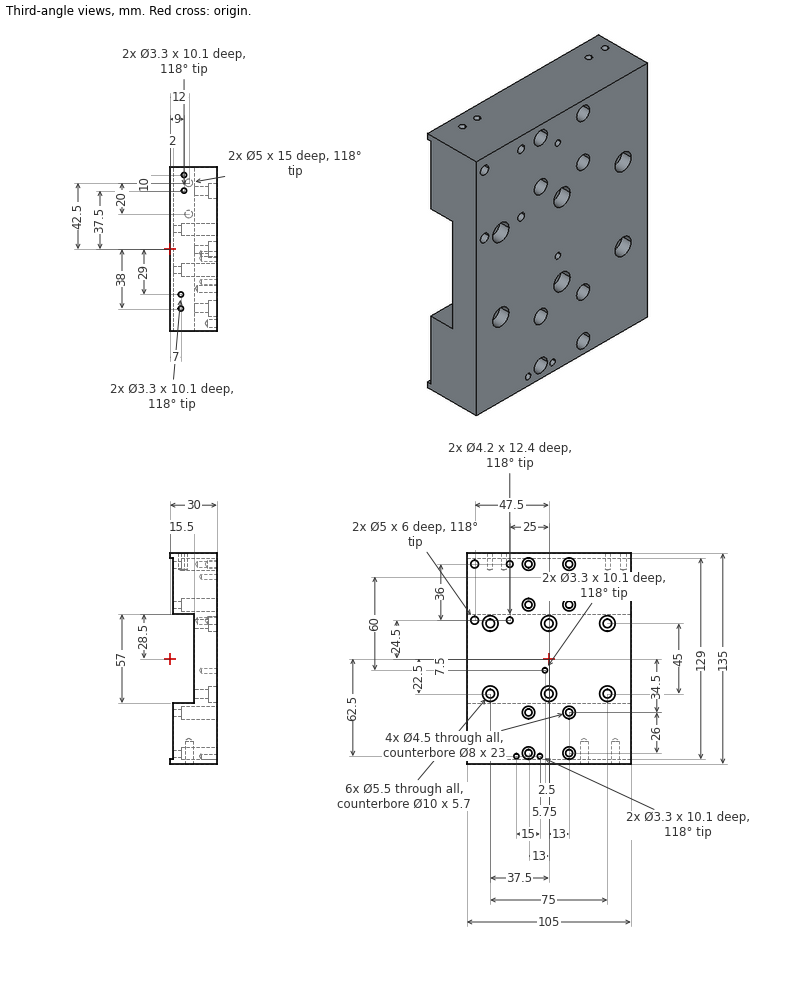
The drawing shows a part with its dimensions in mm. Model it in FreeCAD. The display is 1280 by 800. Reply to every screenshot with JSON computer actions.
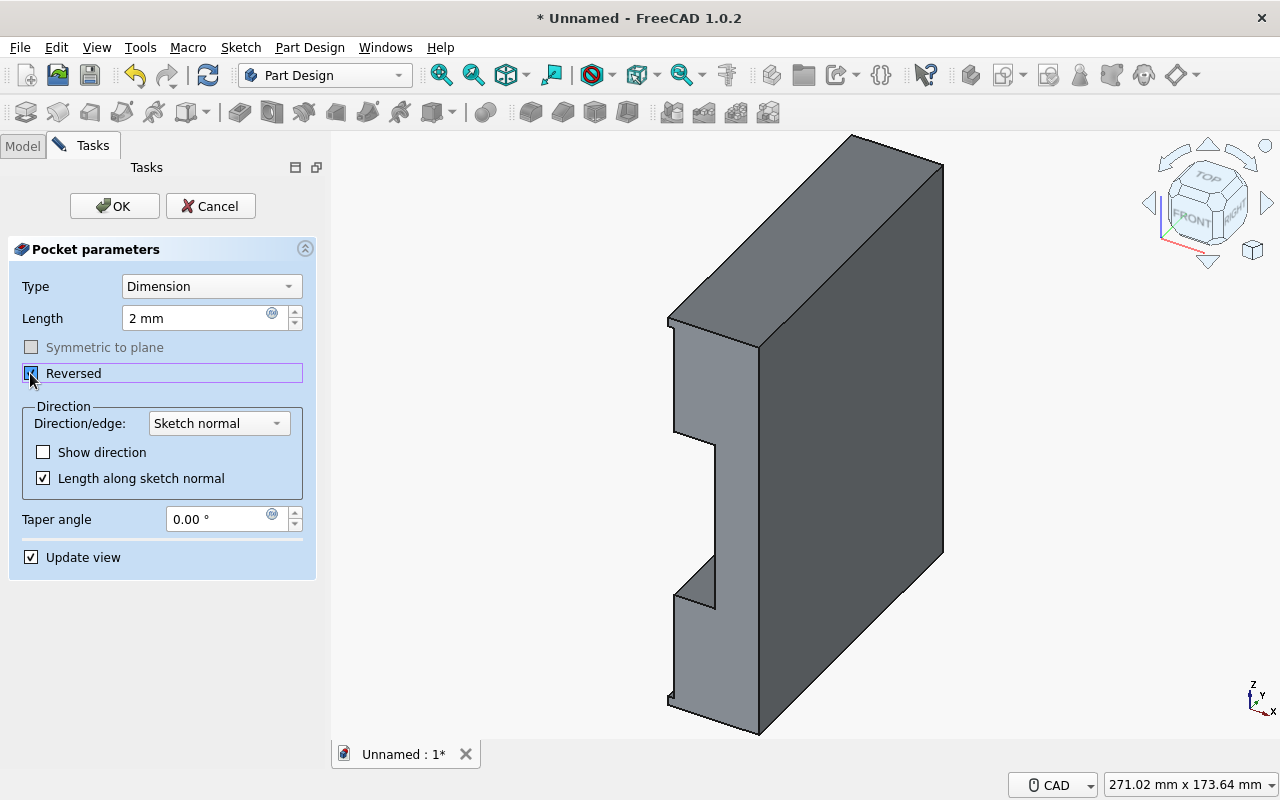
{"action": "left_click", "coordinate": [115, 206]}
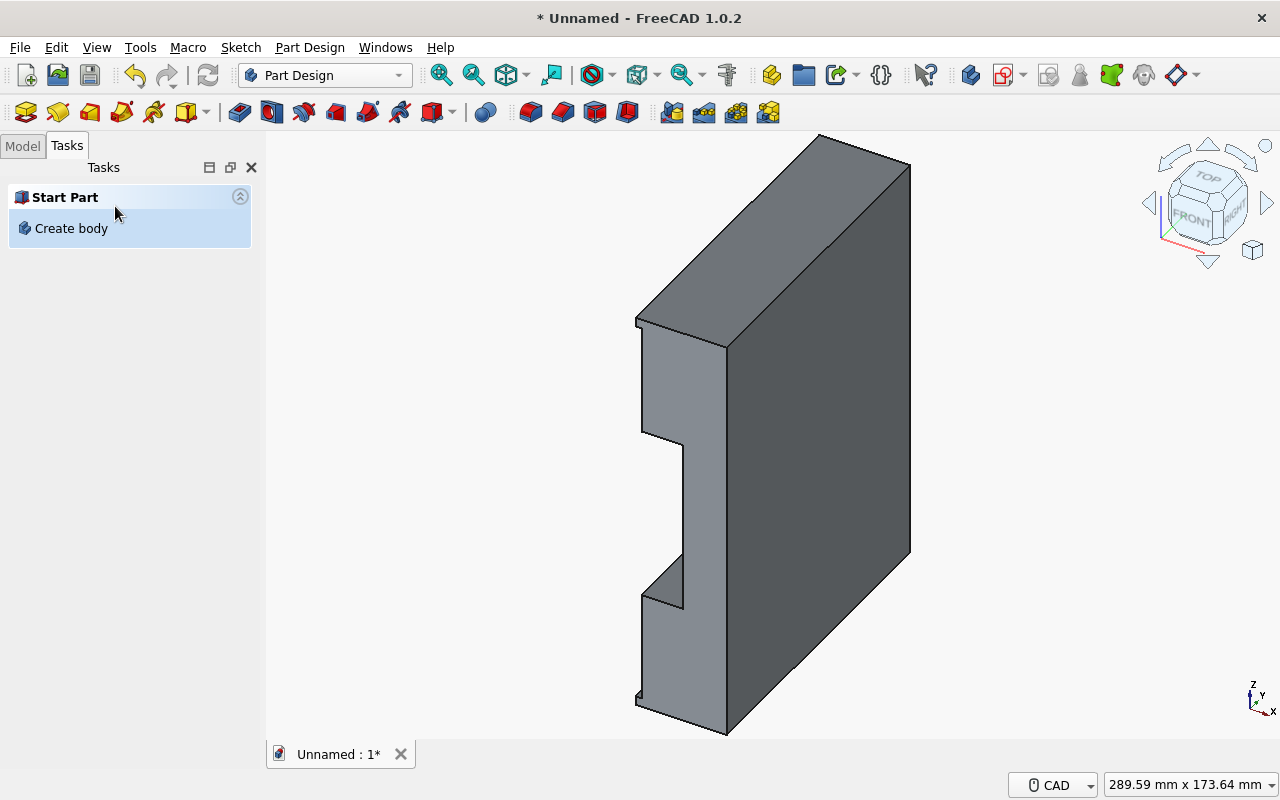
{"action": "left_click", "coordinate": [818, 449]}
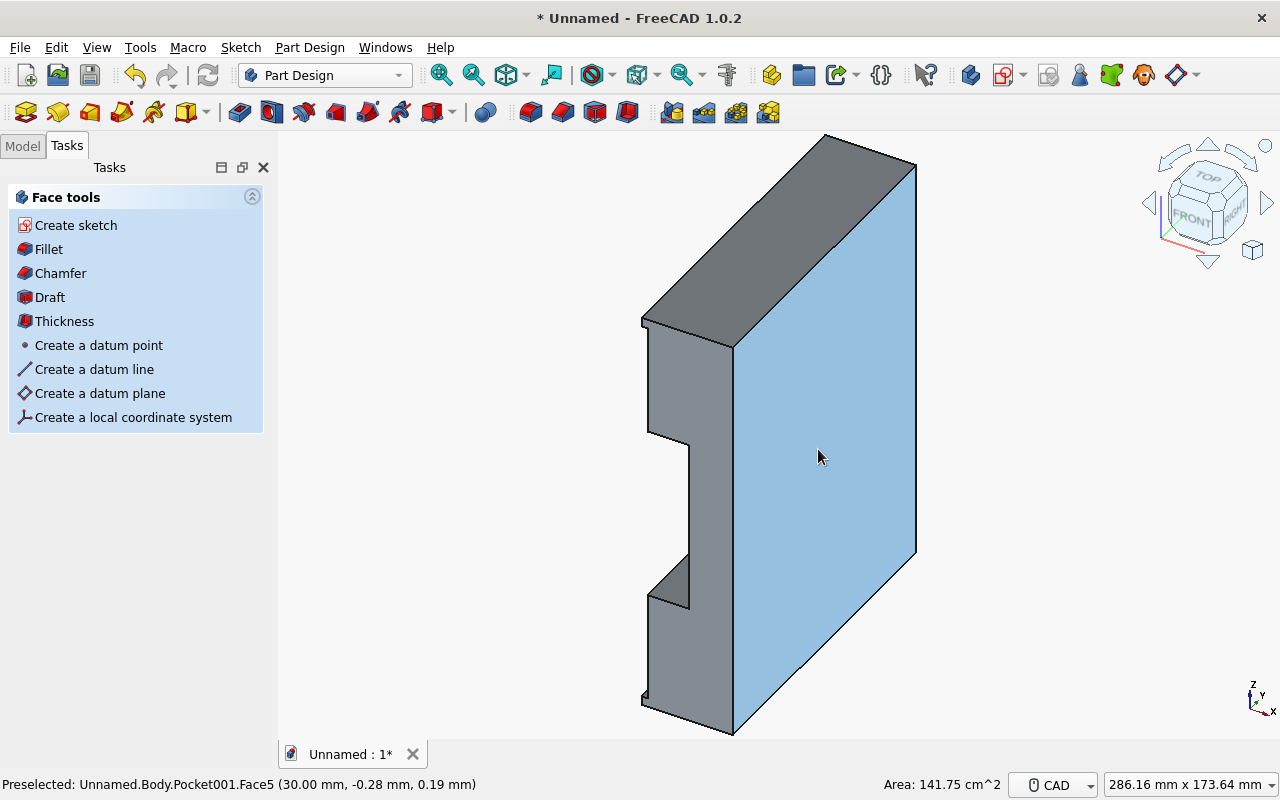
{"action": "left_click", "coordinate": [1004, 76]}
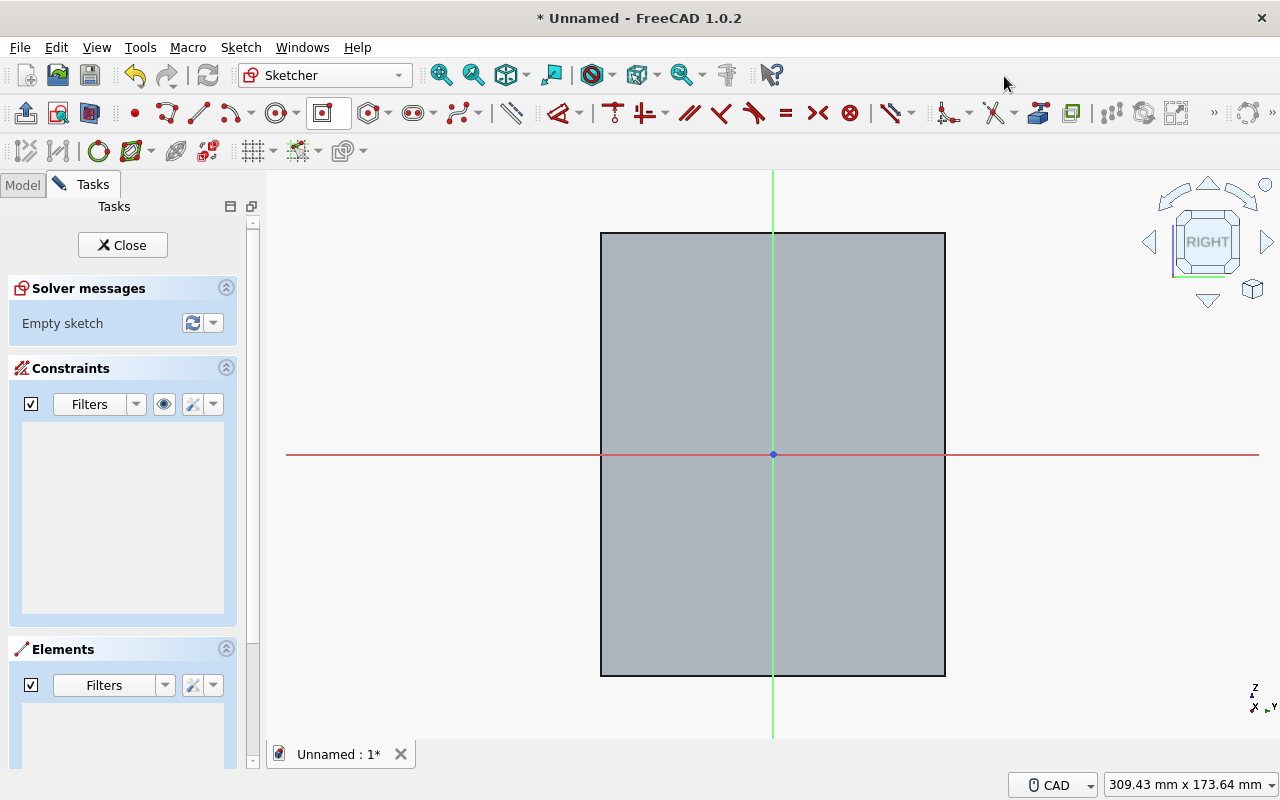
{"action": "scroll", "coordinate": [829, 454], "scroll_direction": "up", "scroll_amount": 4}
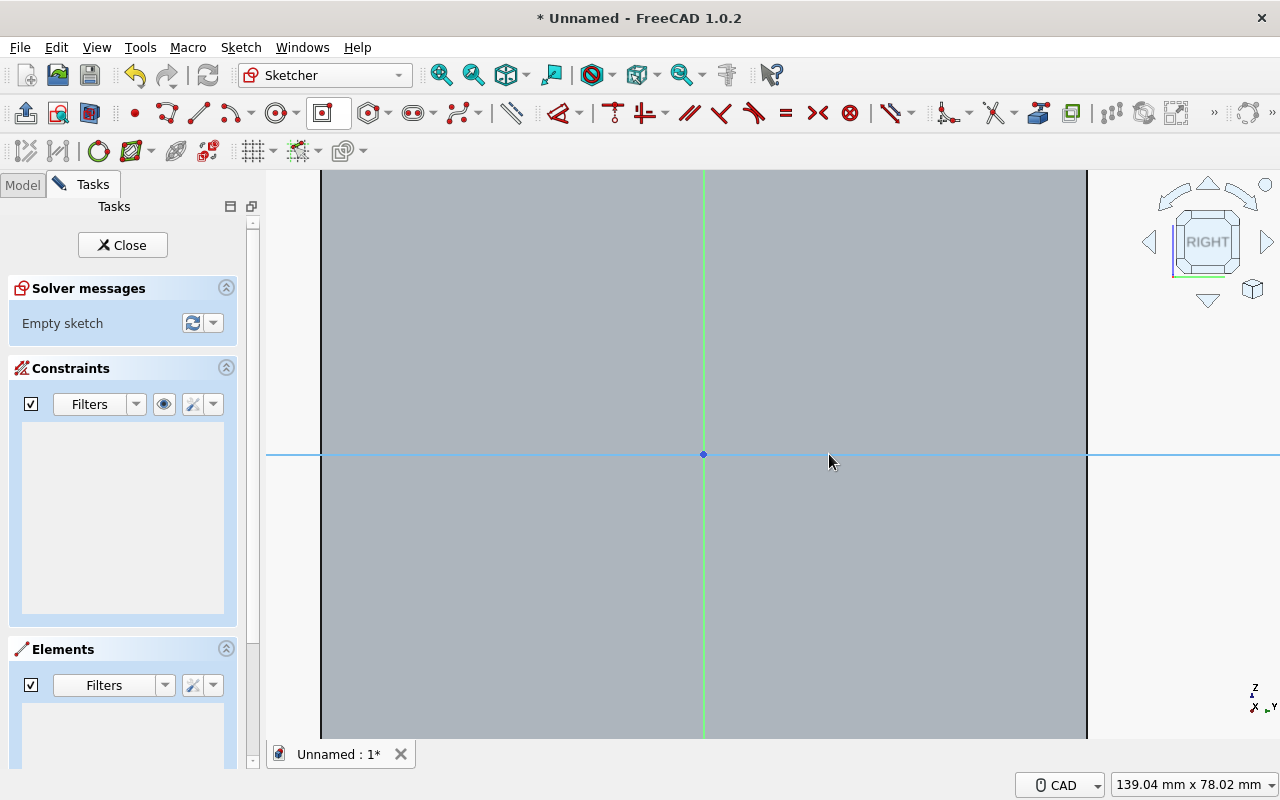
{"action": "left_click", "coordinate": [276, 114]}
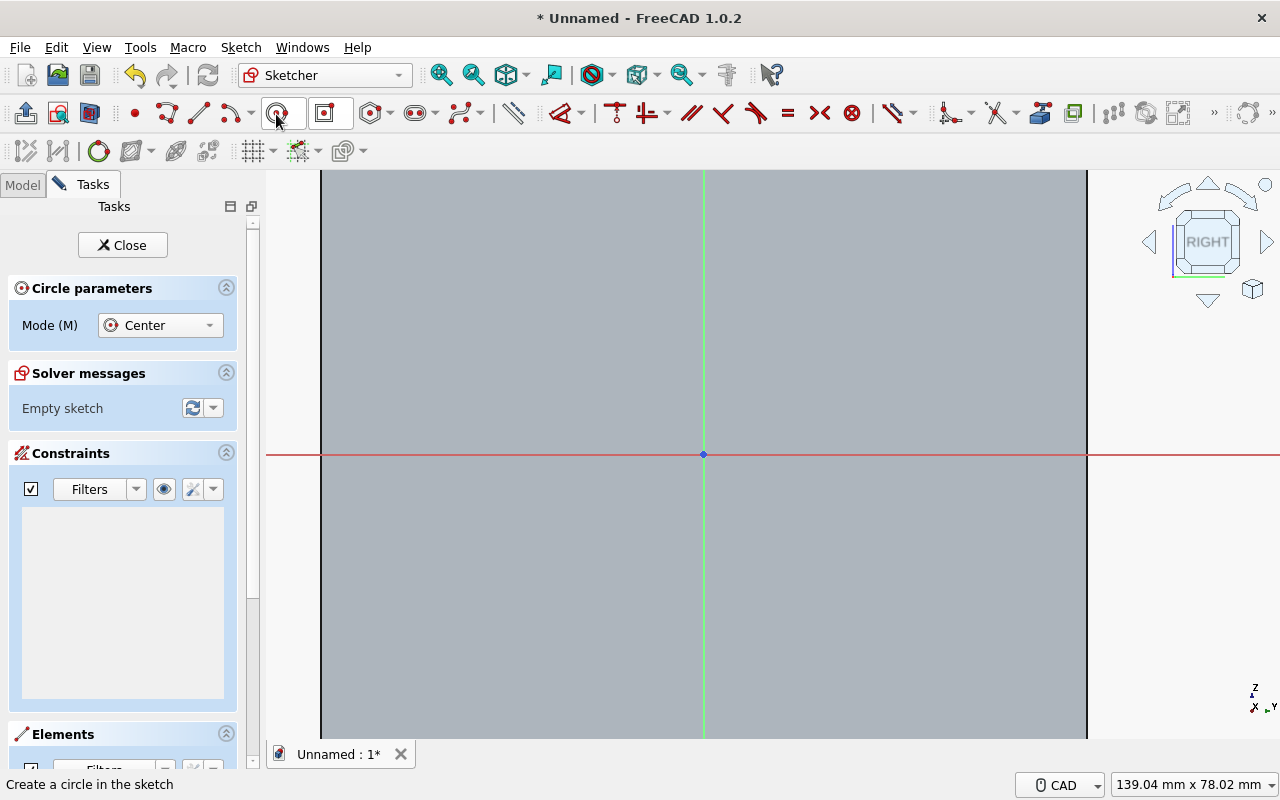
{"action": "left_click", "coordinate": [430, 619]}
{"action": "left_click", "coordinate": [444, 604]}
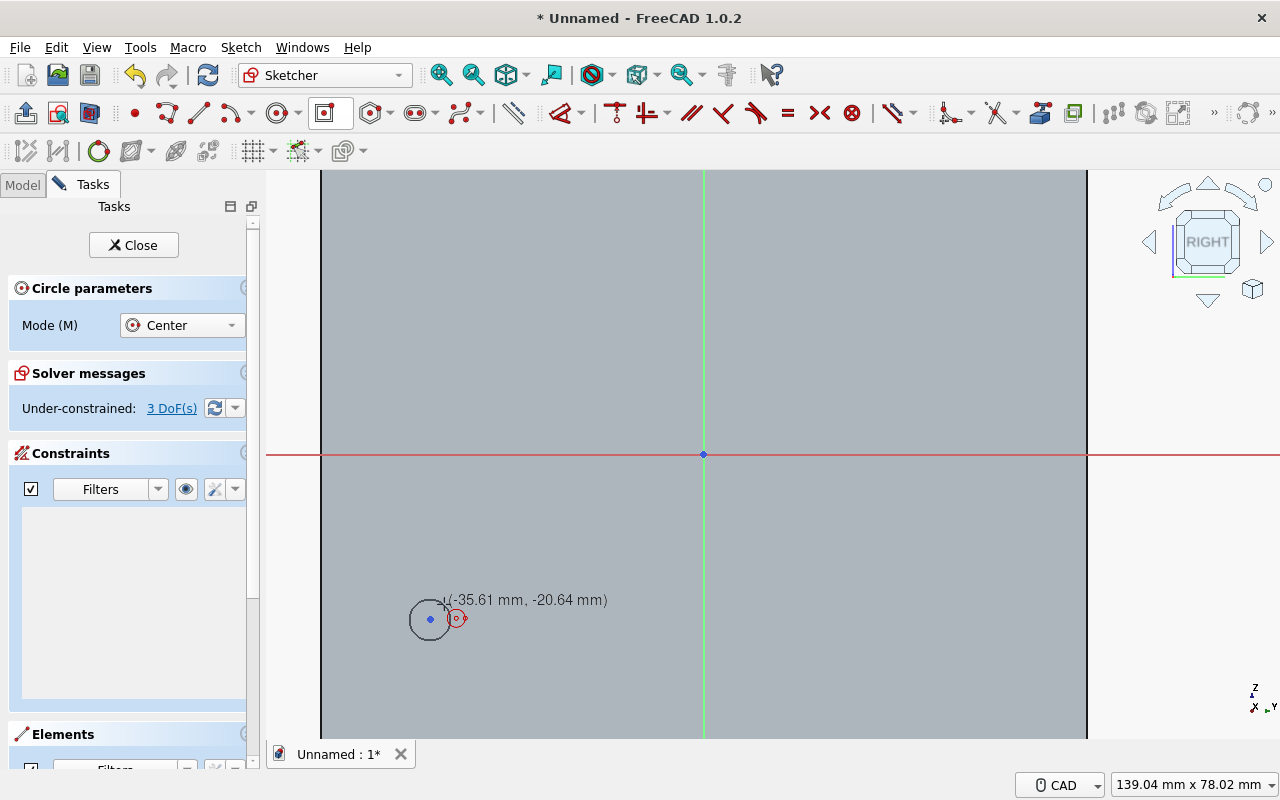
{"action": "left_click", "coordinate": [977, 619]}
{"action": "left_click", "coordinate": [991, 604]}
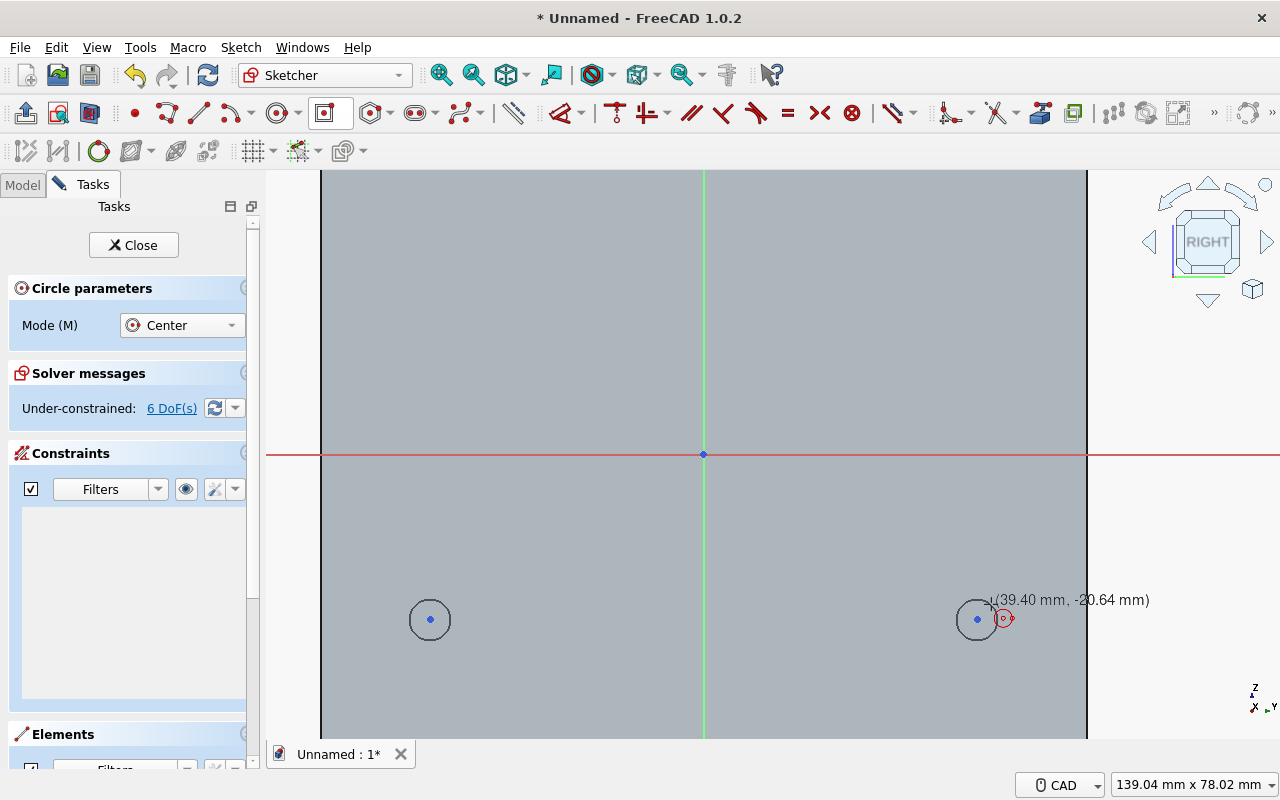
{"action": "left_click", "coordinate": [977, 290]}
{"action": "left_click", "coordinate": [991, 276]}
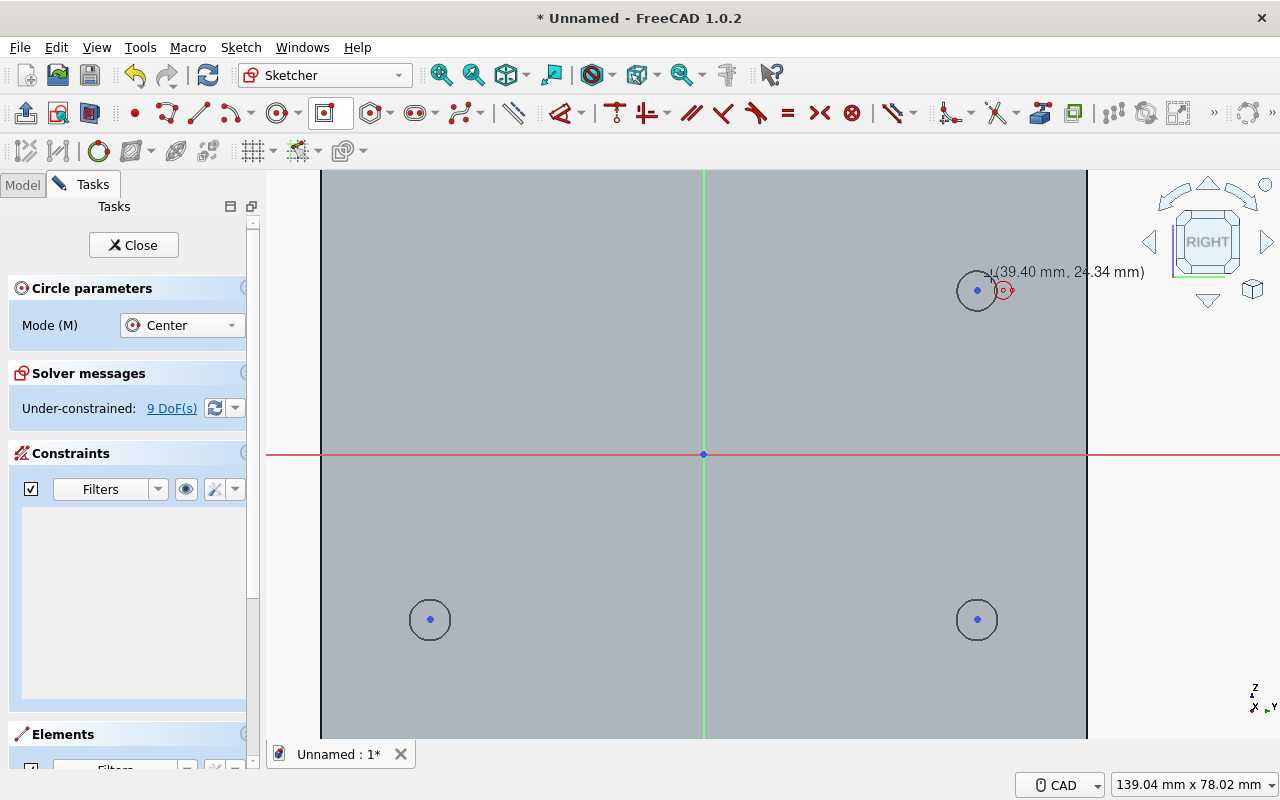
{"action": "left_click", "coordinate": [704, 290]}
{"action": "left_click", "coordinate": [718, 276]}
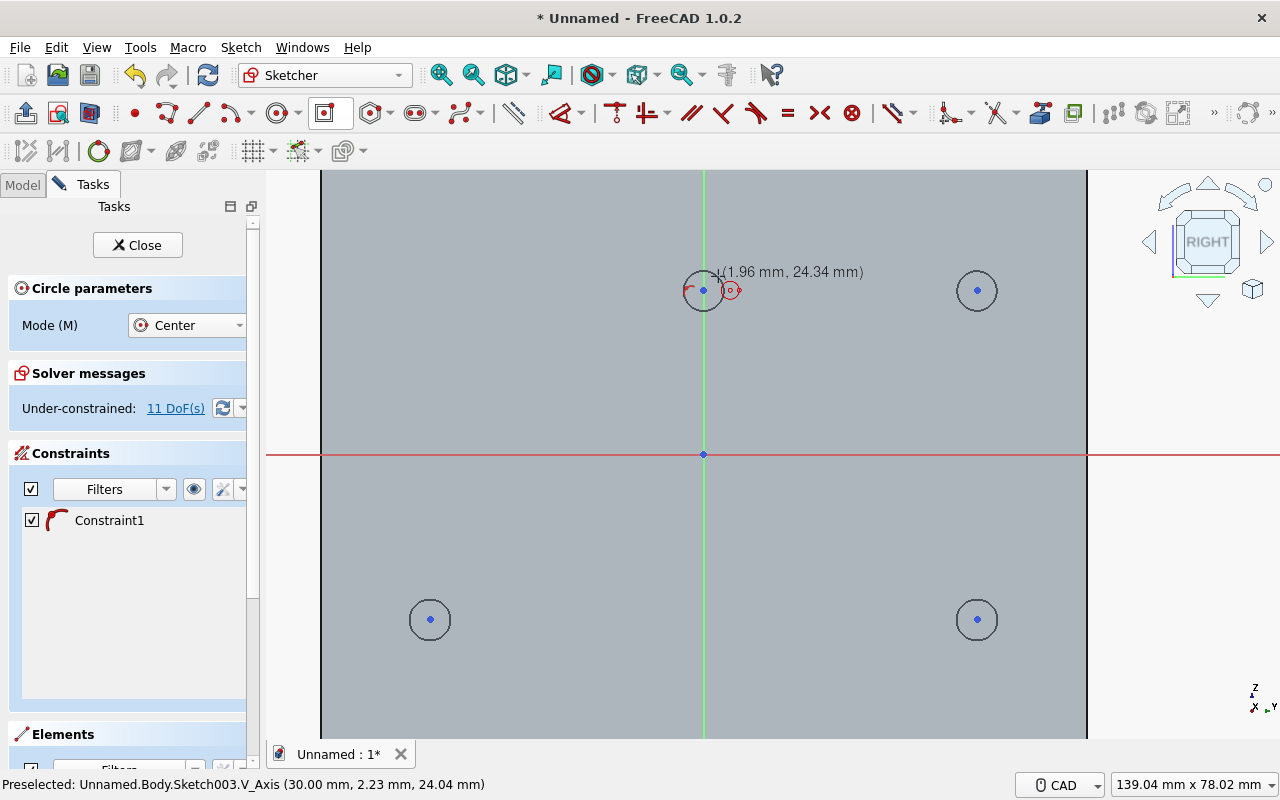
{"action": "left_click", "coordinate": [704, 619]}
{"action": "left_click", "coordinate": [718, 604]}